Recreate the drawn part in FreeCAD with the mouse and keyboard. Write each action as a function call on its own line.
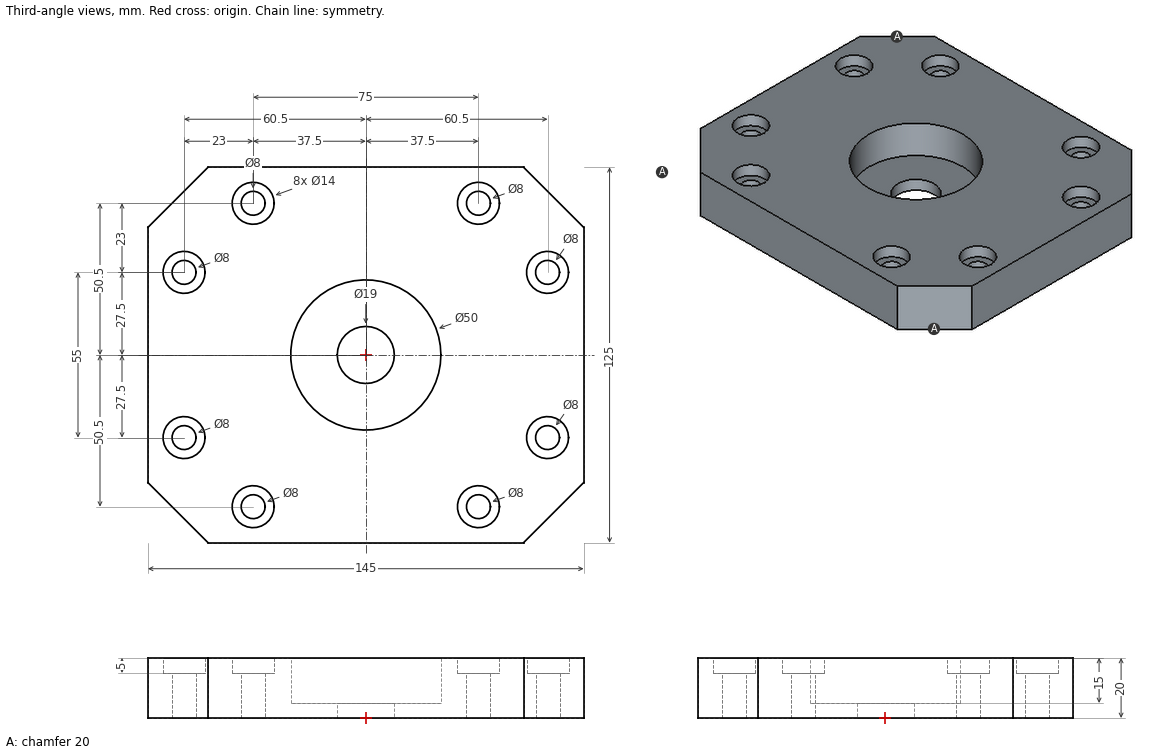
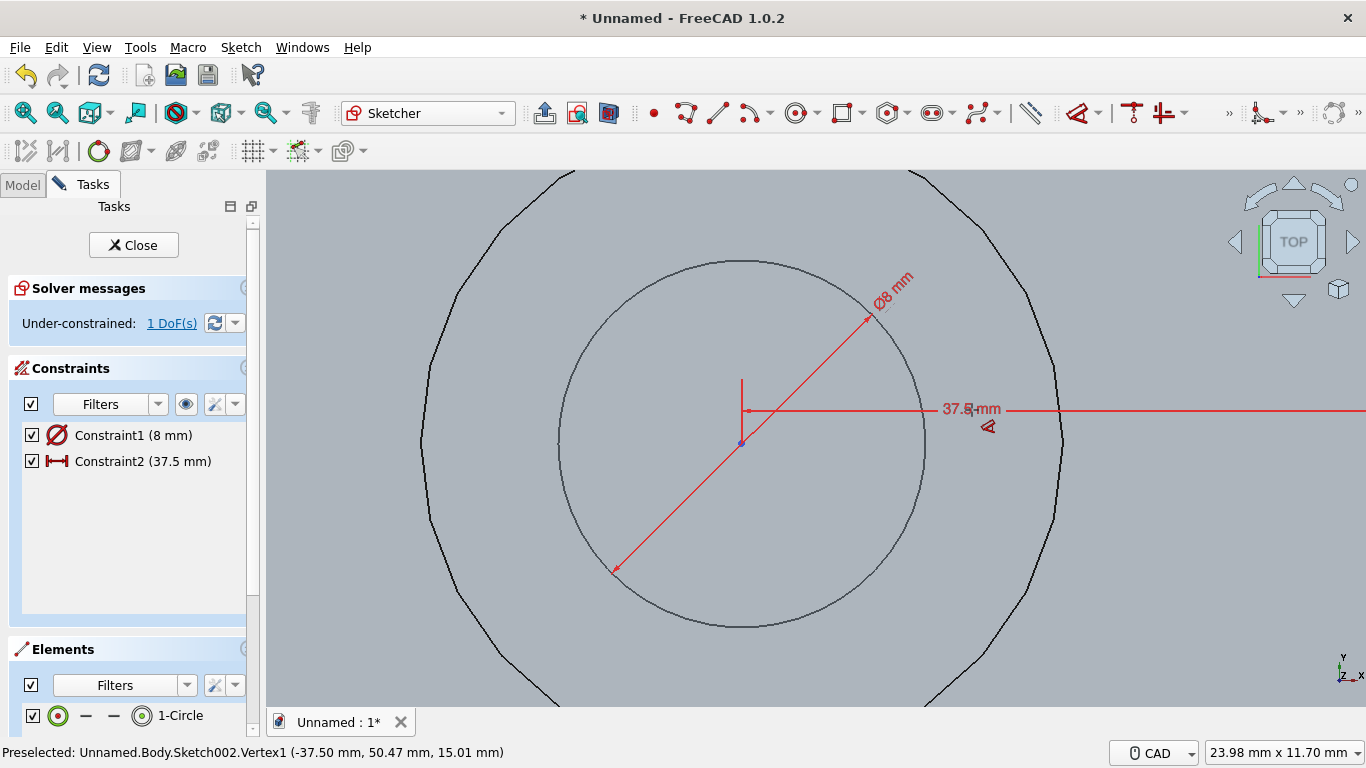
click(742, 444)
click(708, 562)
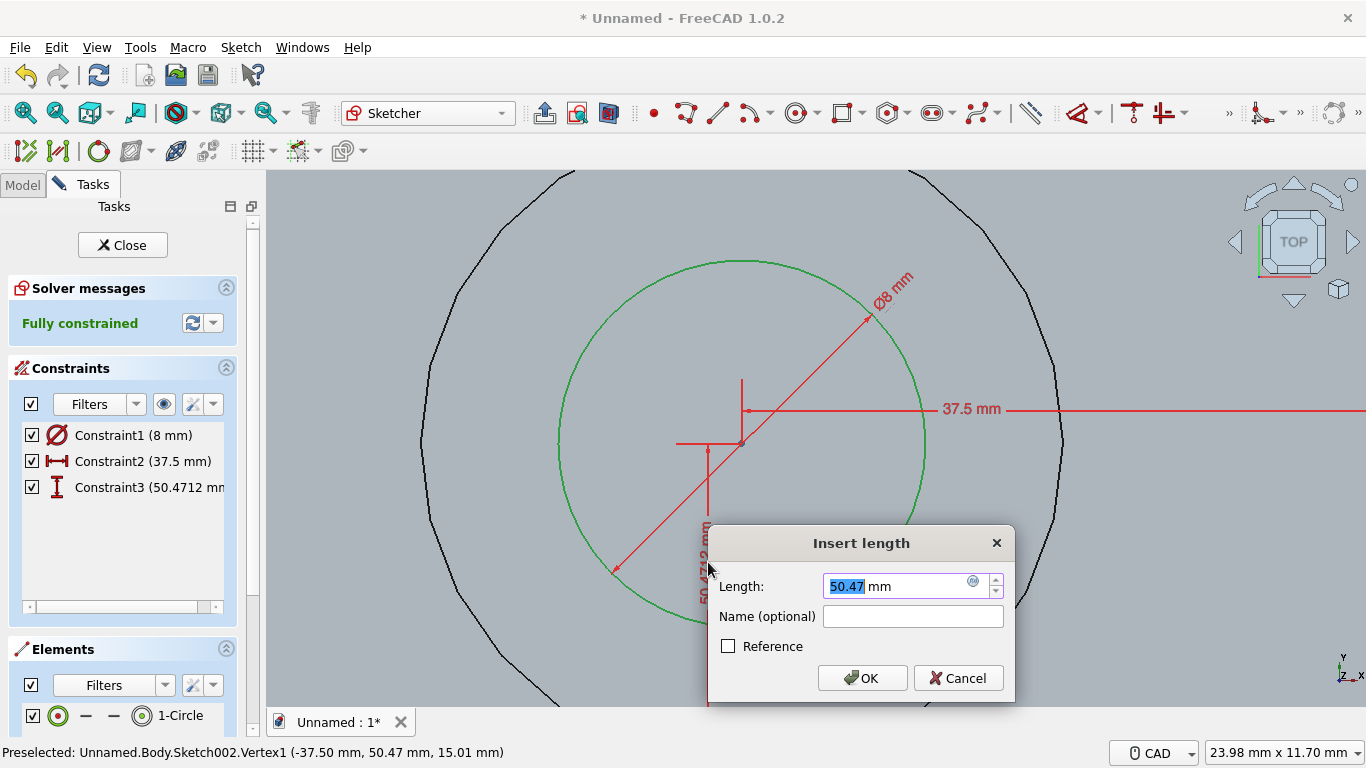
text(50.5)
key(Return)
key(Escape)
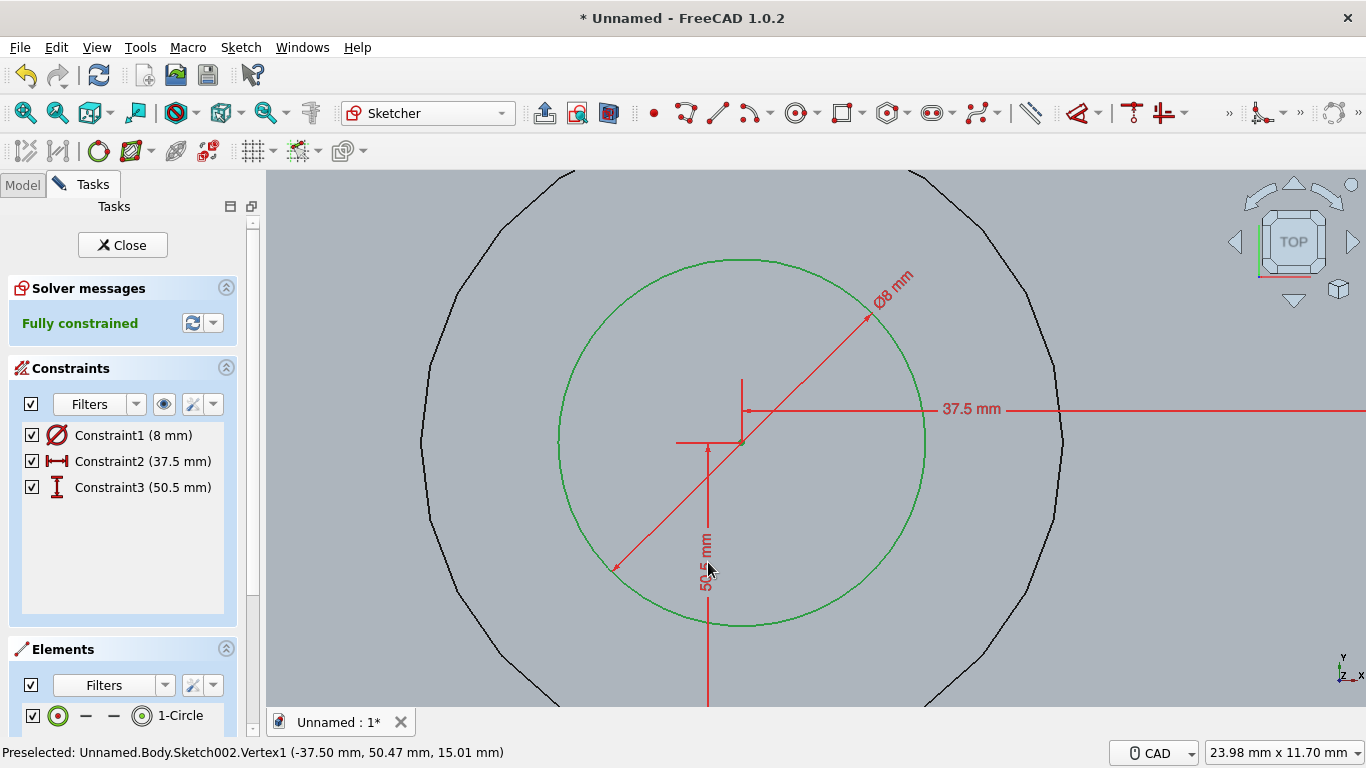
click(123, 245)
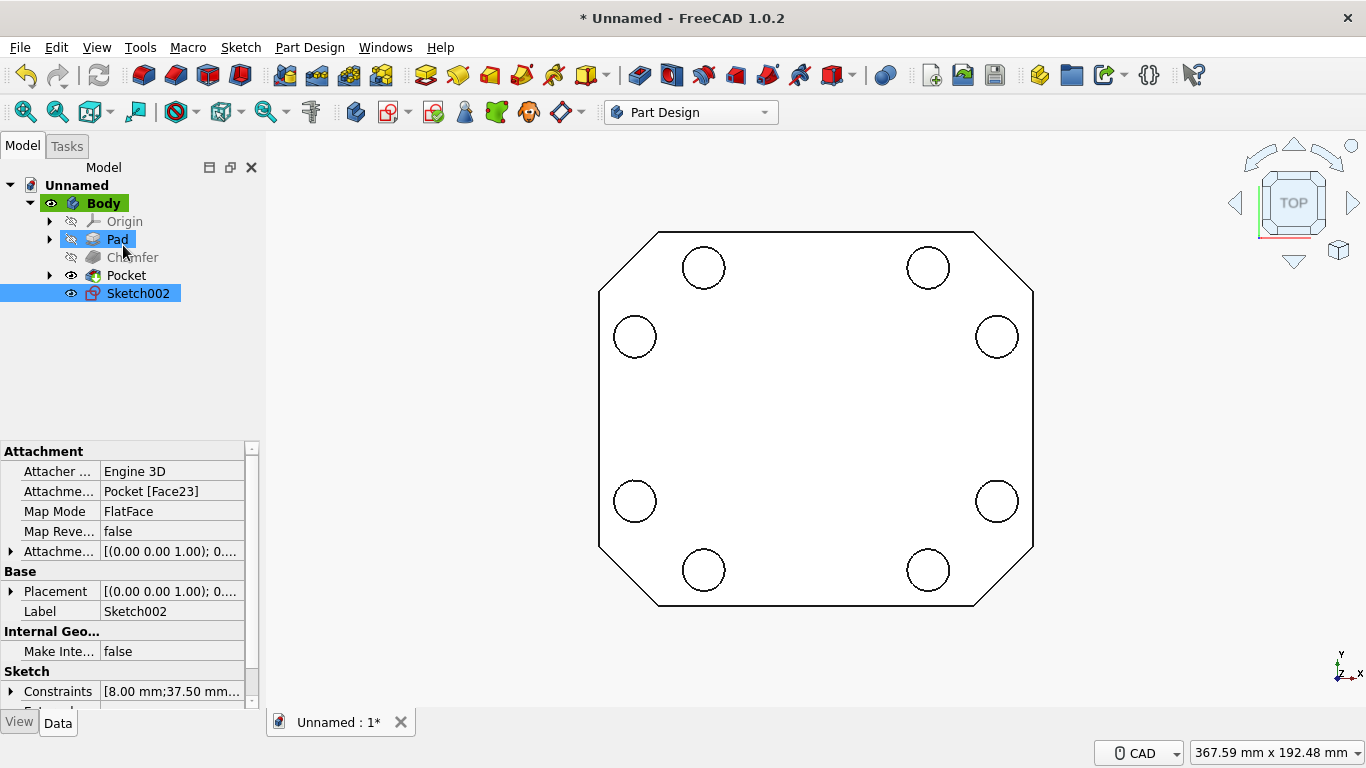
click(640, 76)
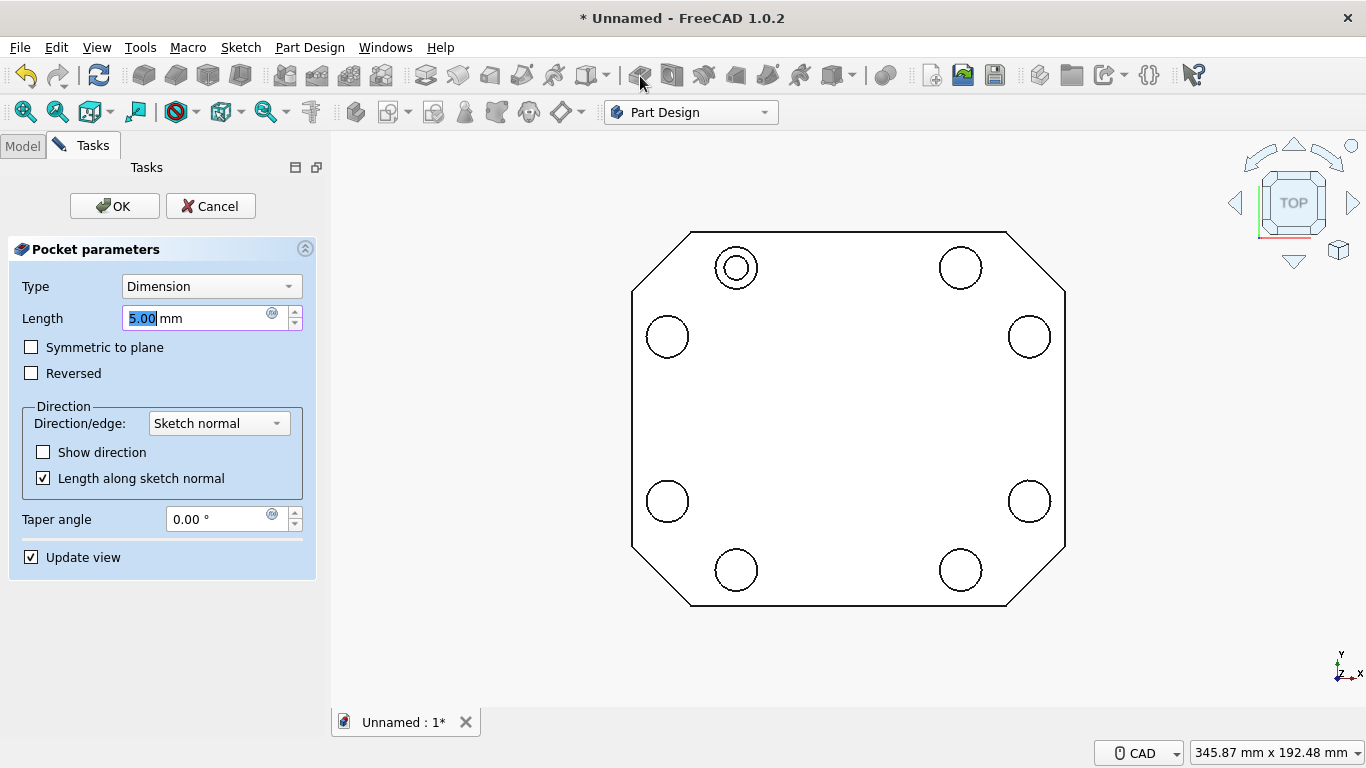
click(212, 286)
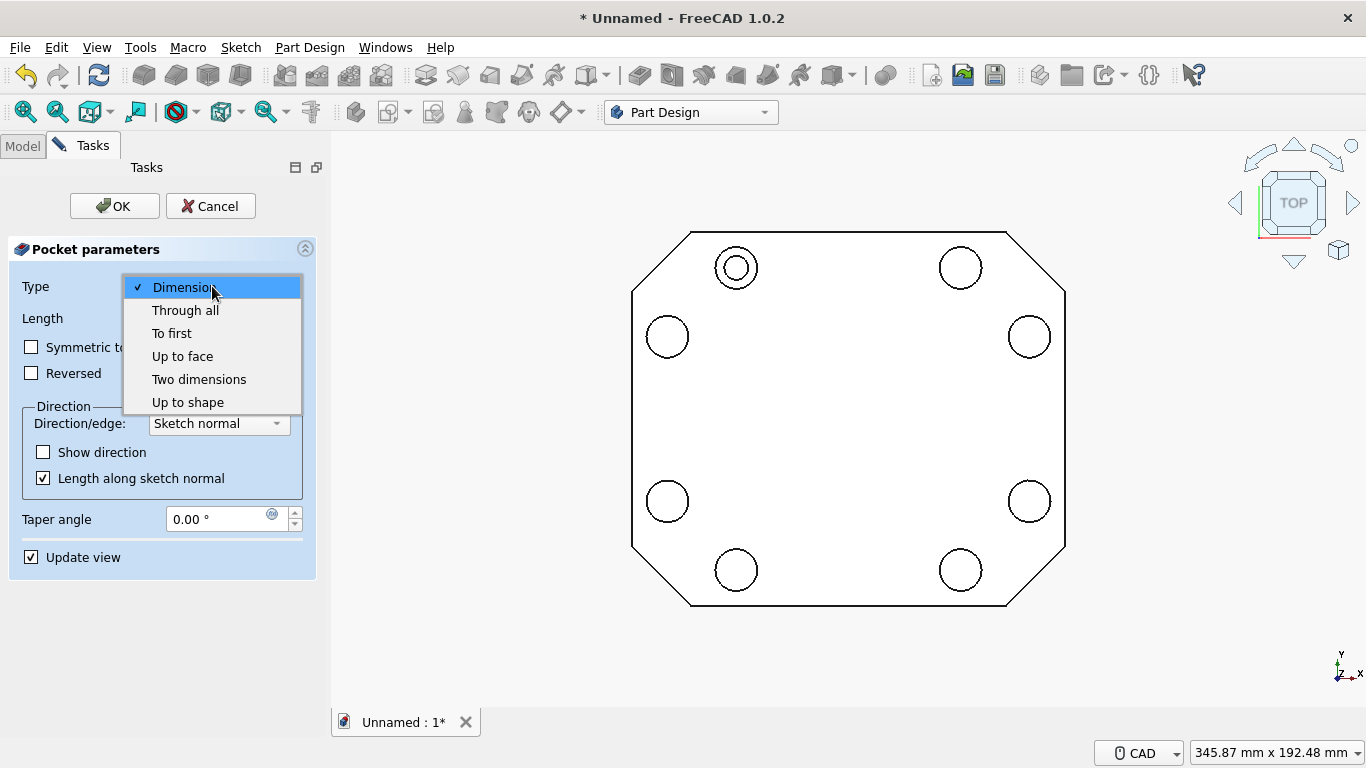
click(212, 334)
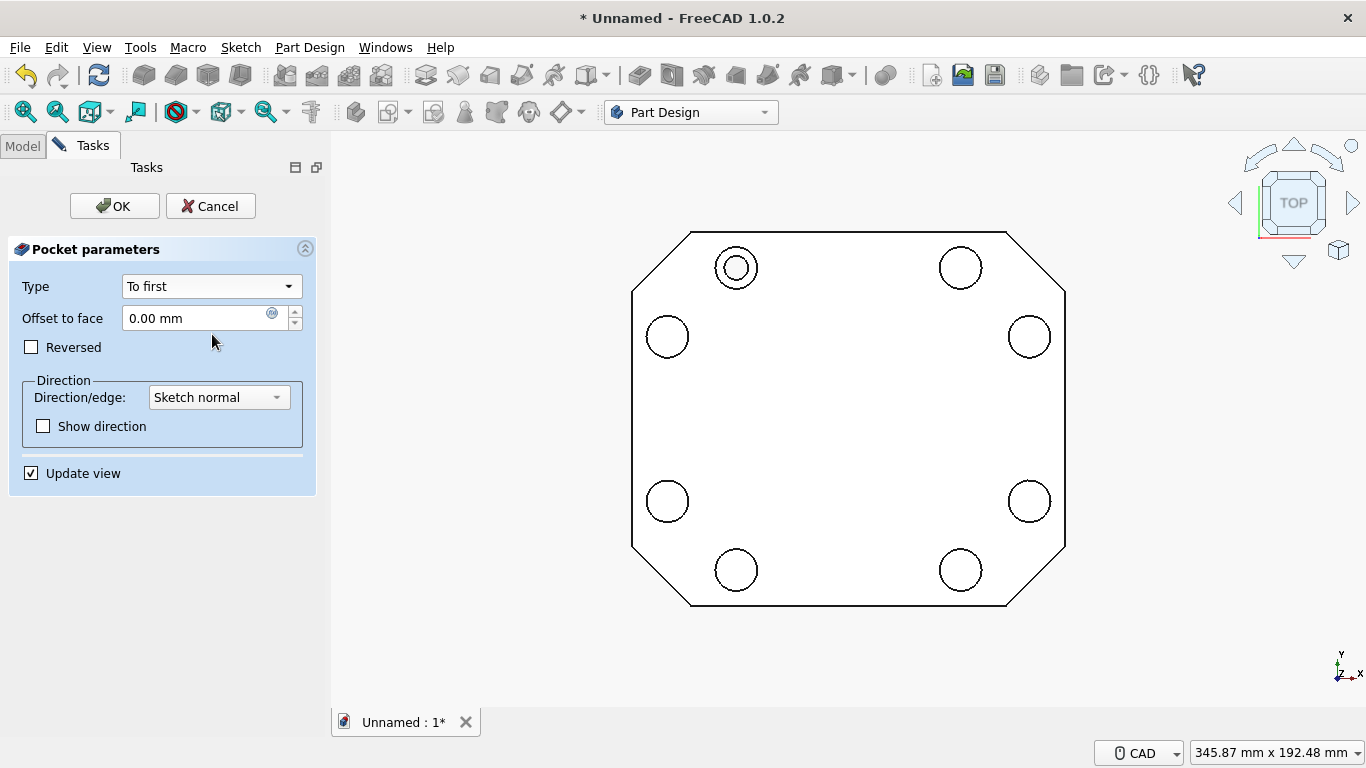
click(115, 206)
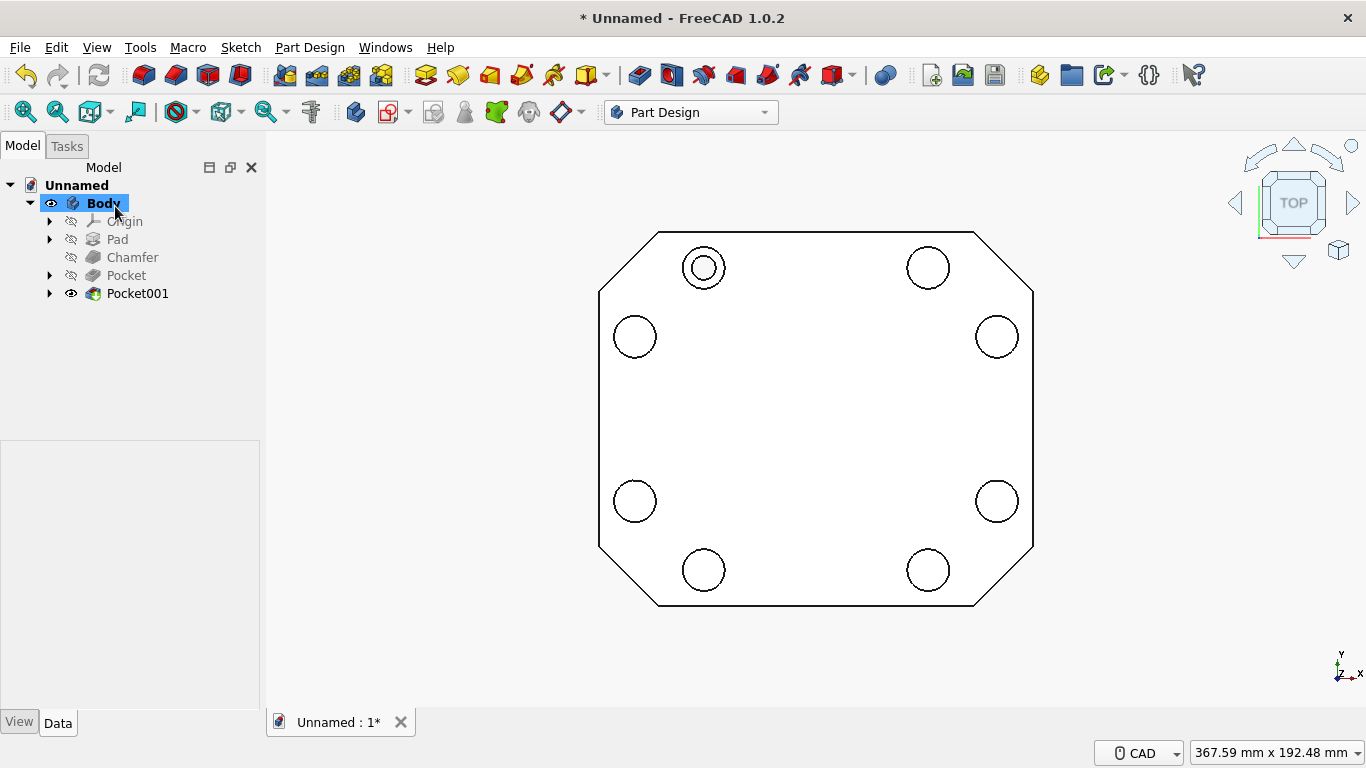
click(635, 336)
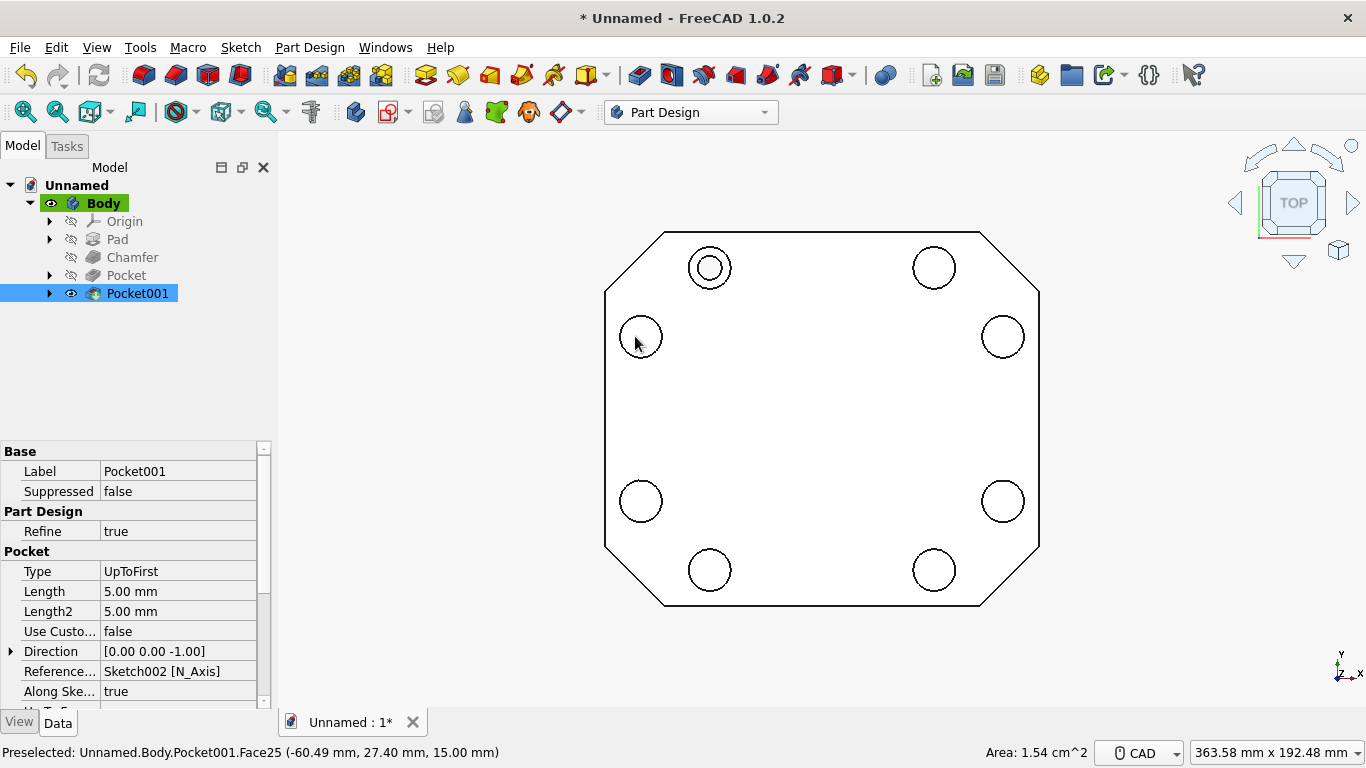
click(388, 112)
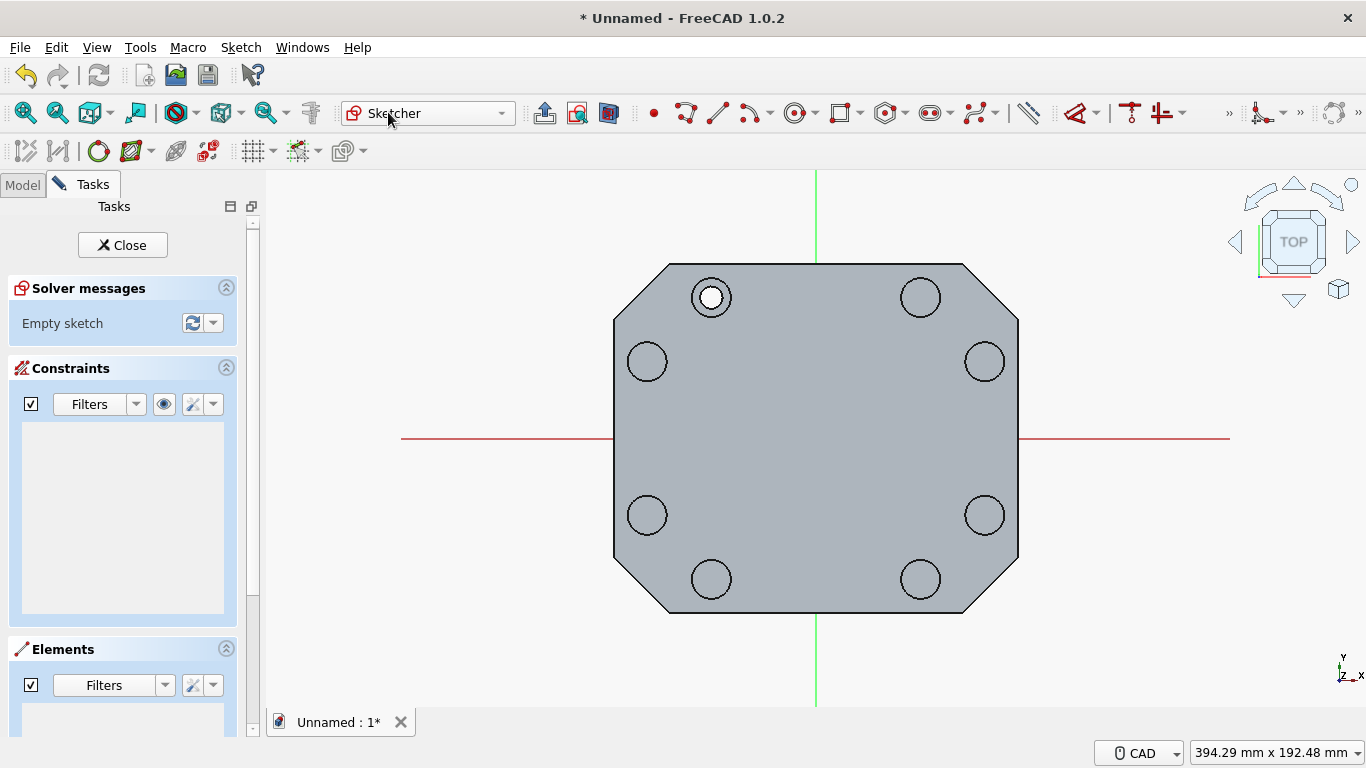
scroll(641, 357, up, 14)